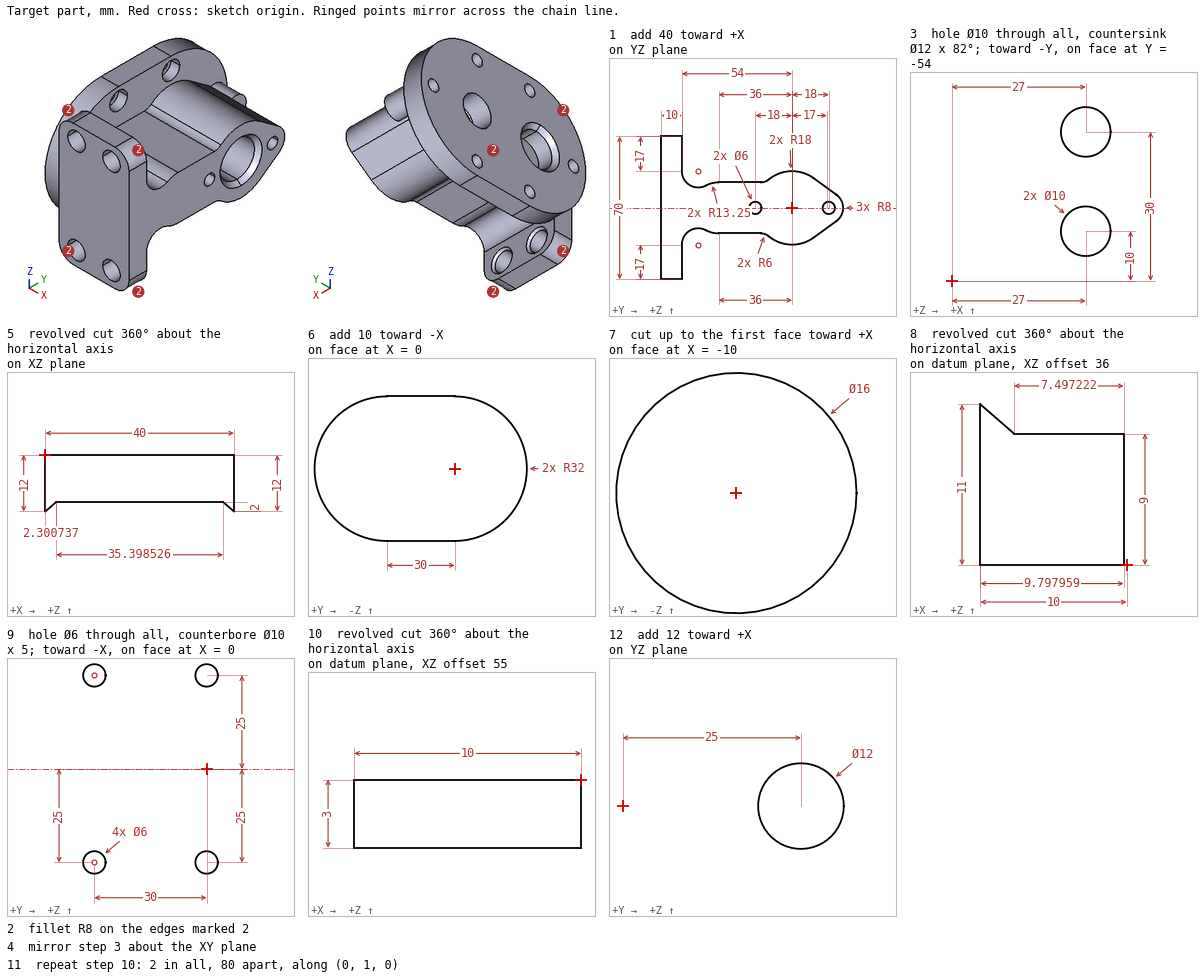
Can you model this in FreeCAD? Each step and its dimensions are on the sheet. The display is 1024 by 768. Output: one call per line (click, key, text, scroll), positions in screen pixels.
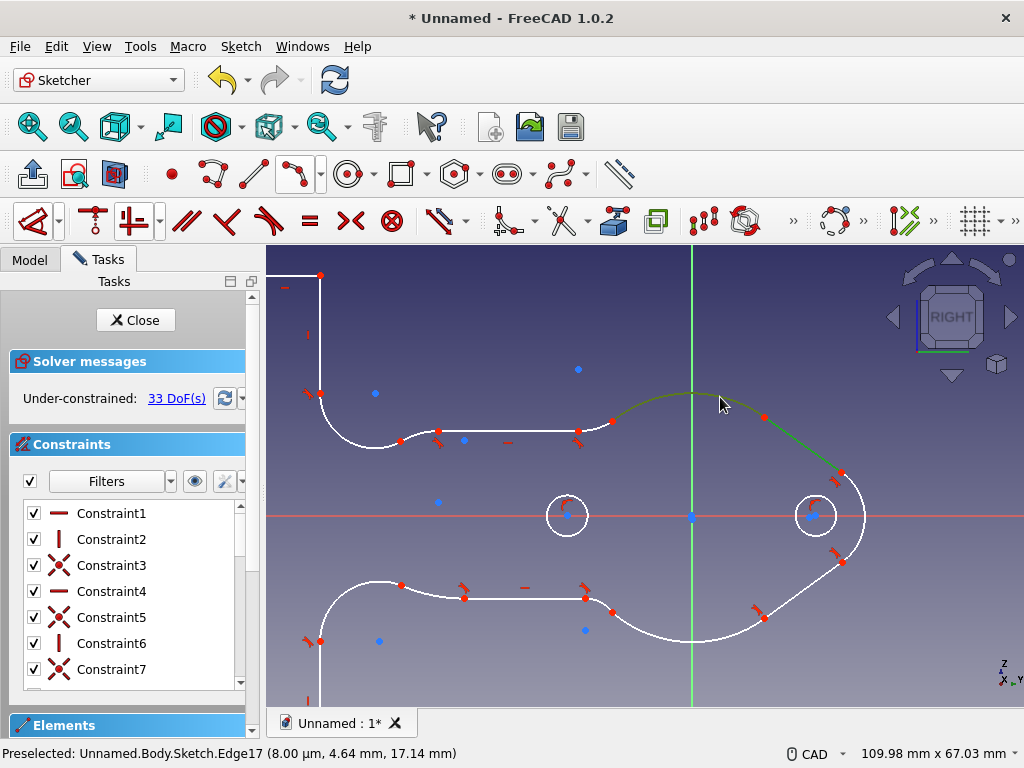
click(269, 222)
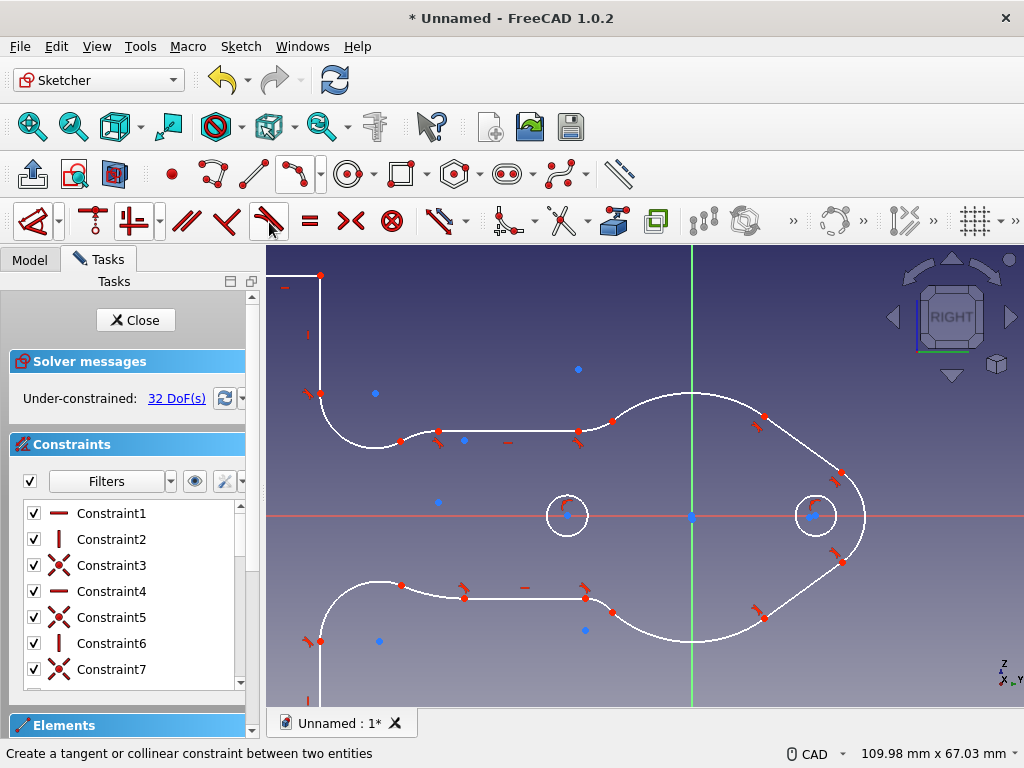
click(427, 432)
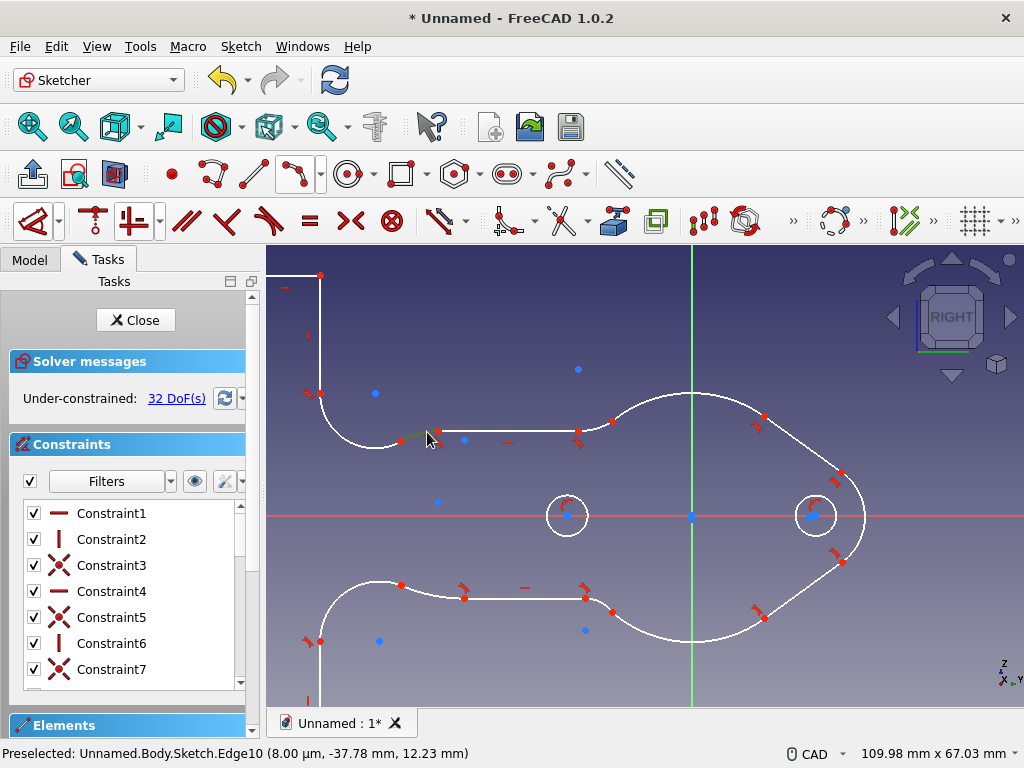
click(330, 425)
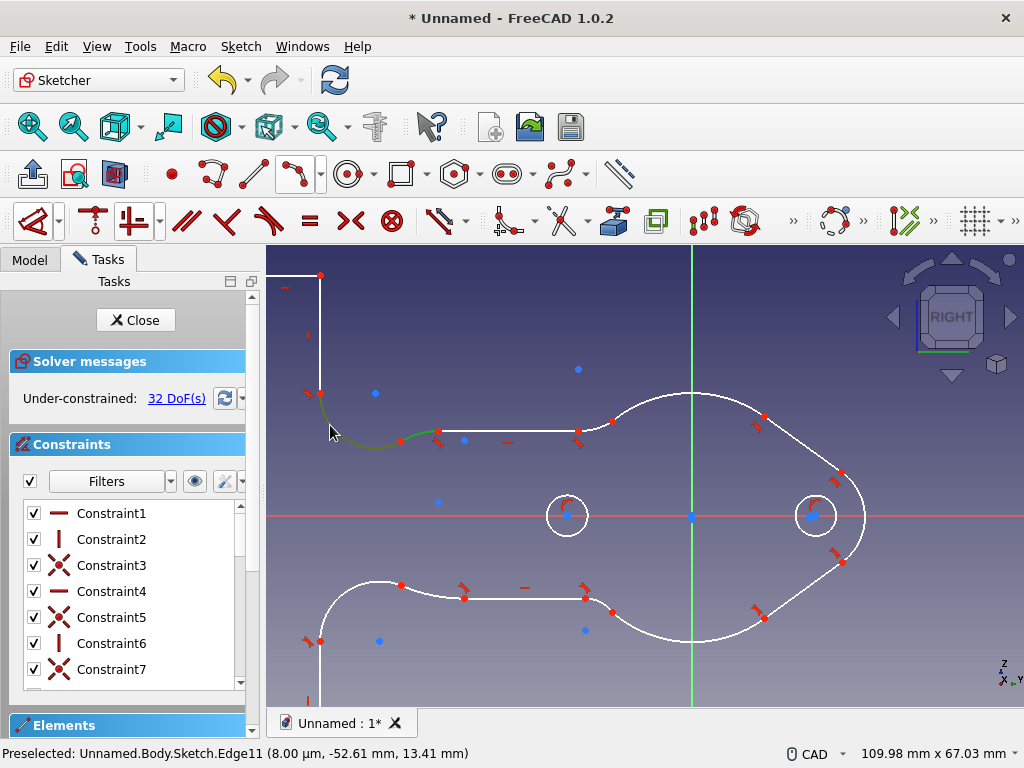
click(269, 222)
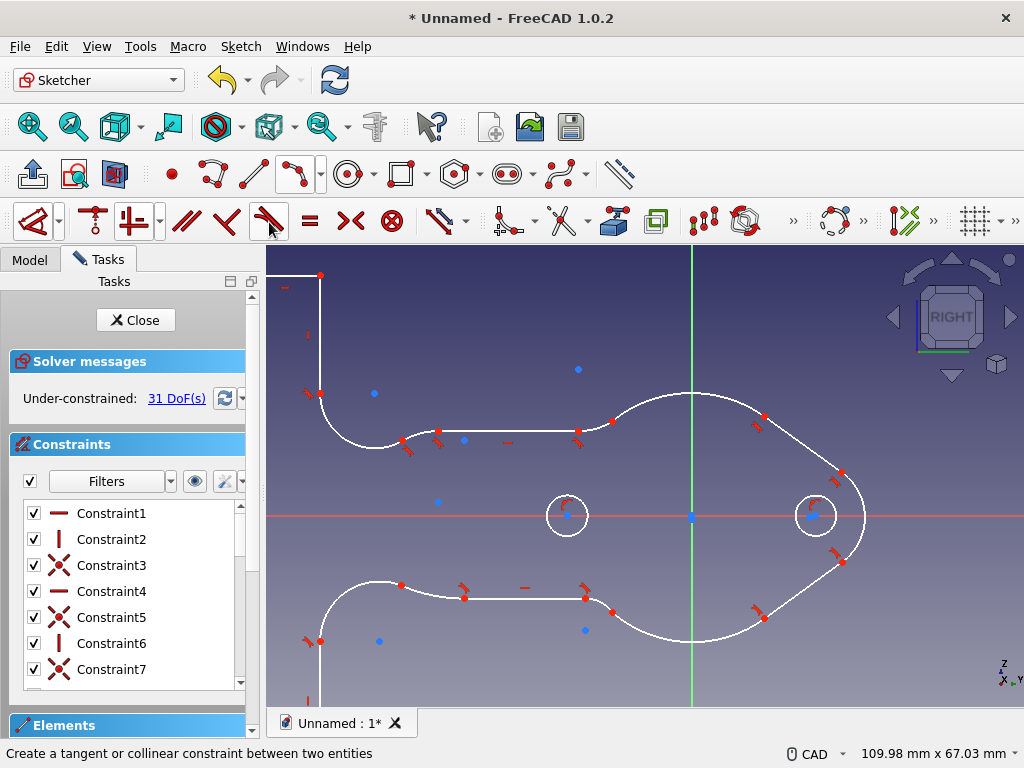
click(367, 583)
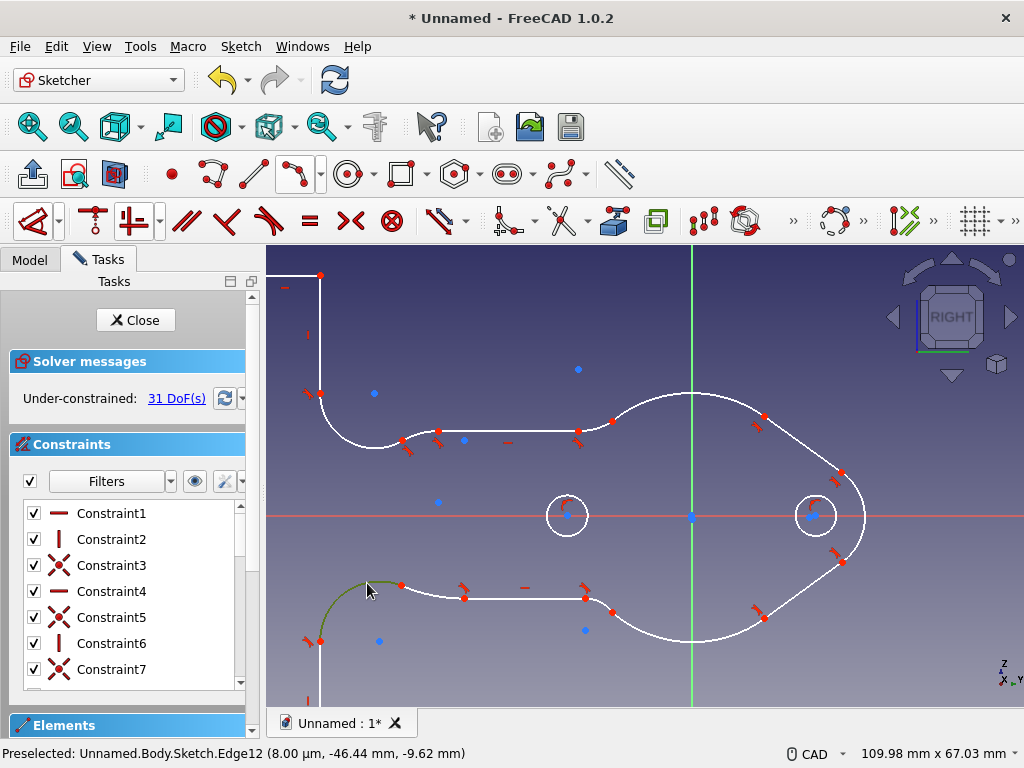
click(419, 592)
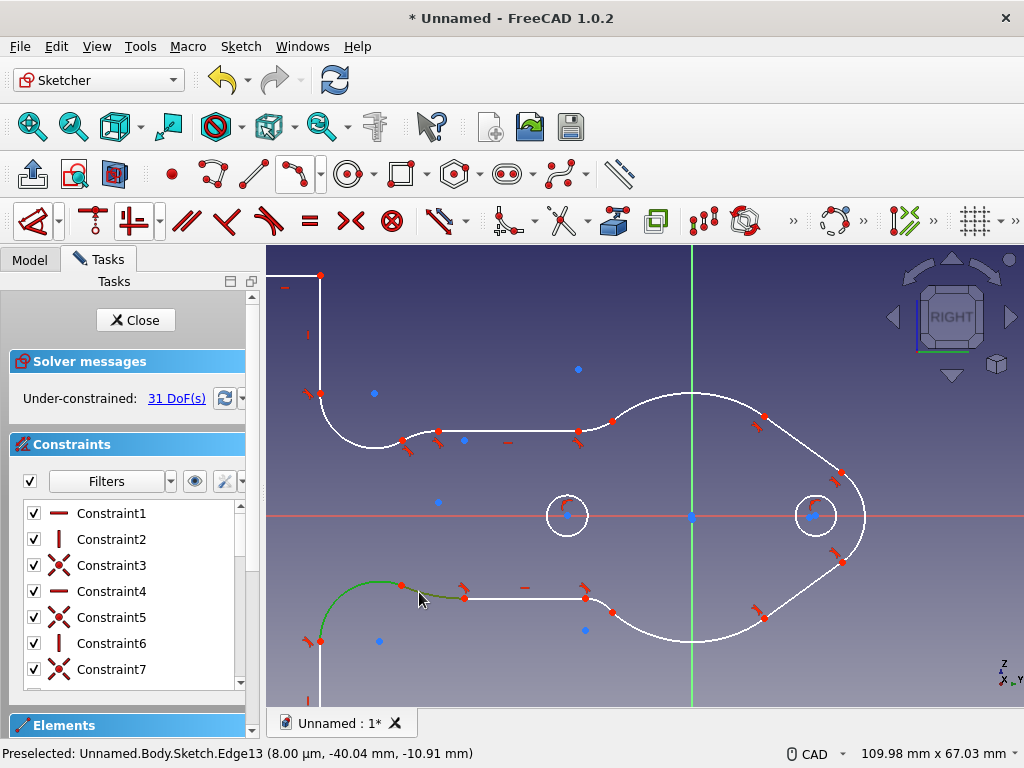
click(269, 222)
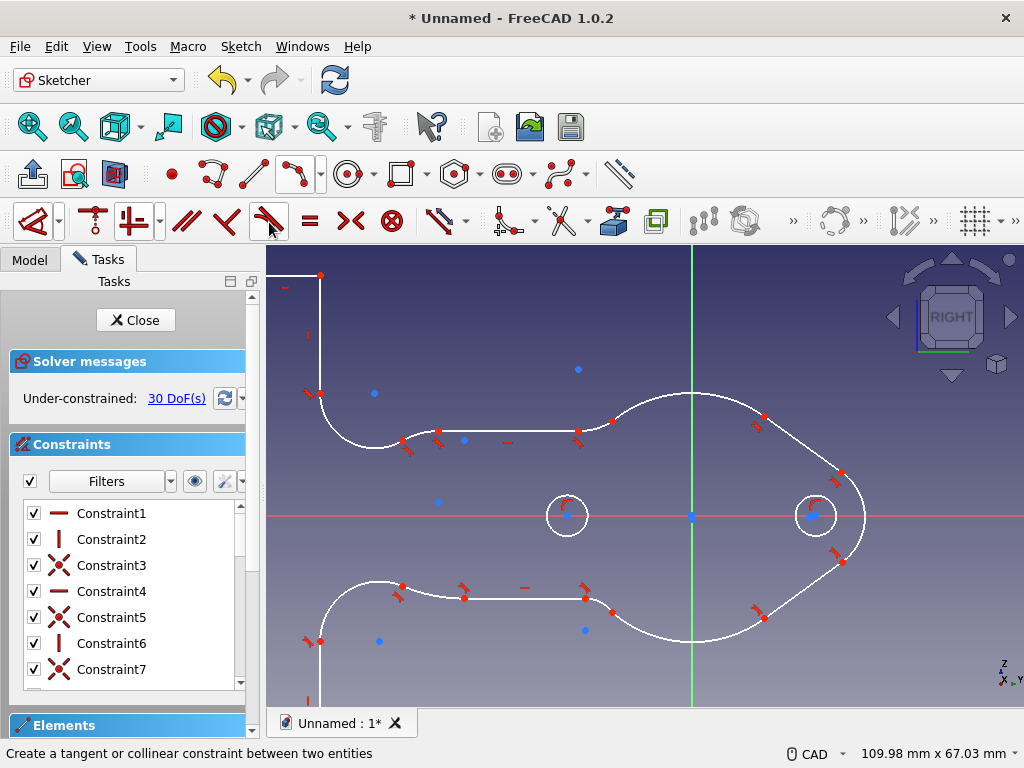
scroll(606, 606, up, 2)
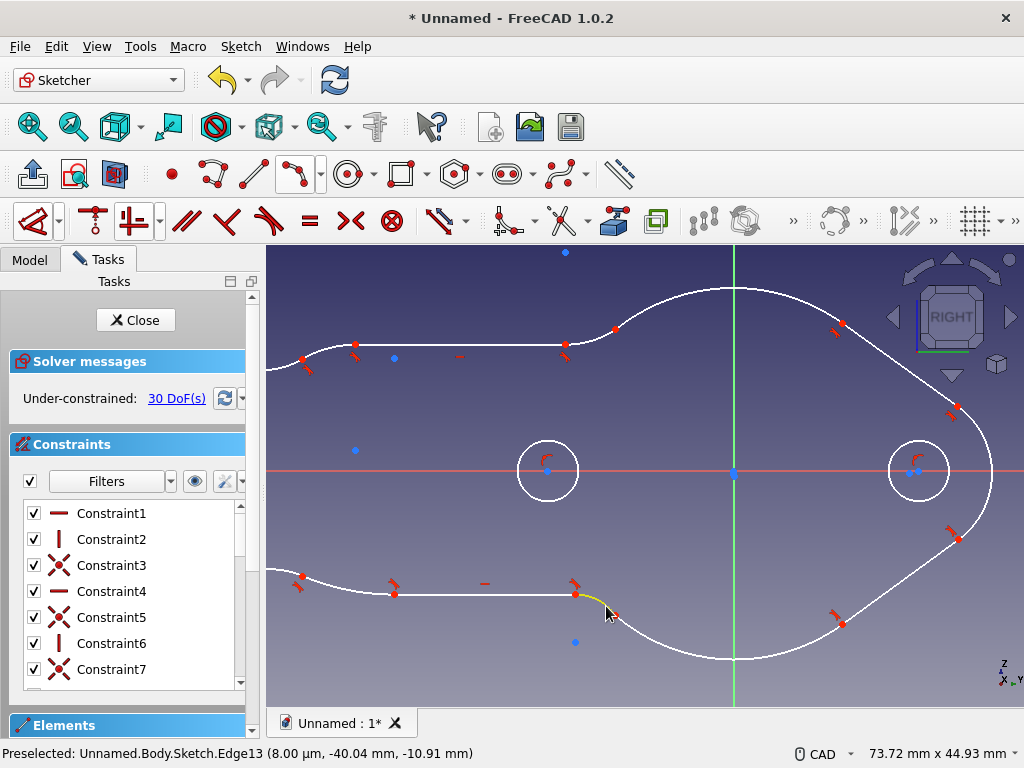
click(606, 605)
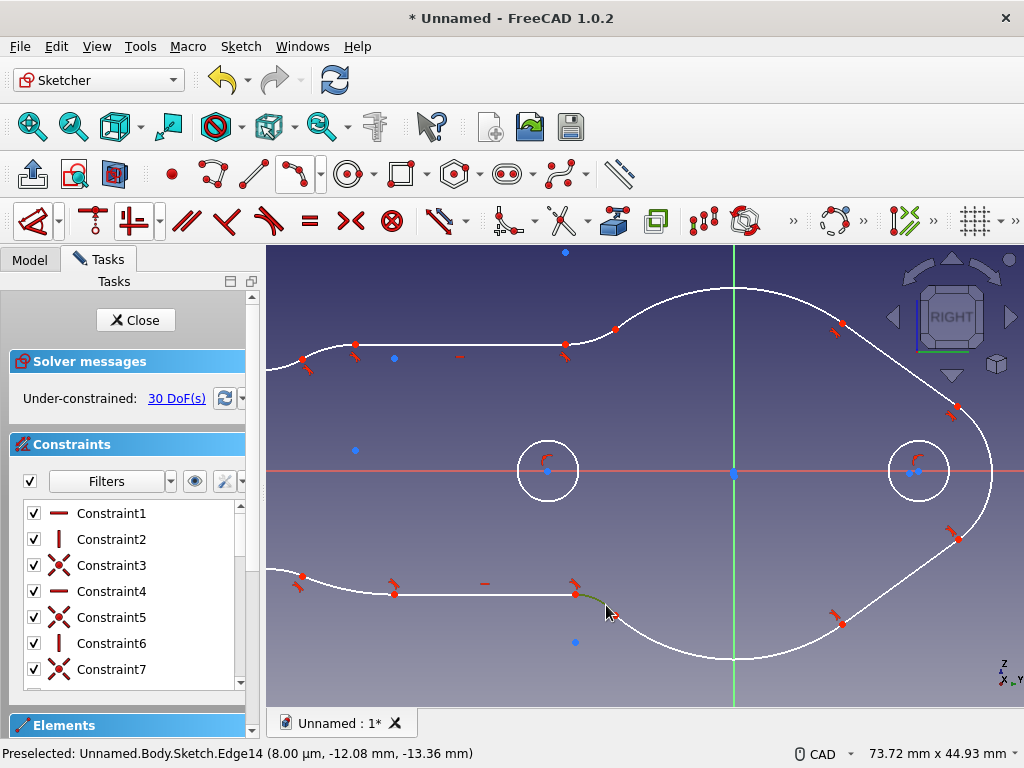
click(679, 651)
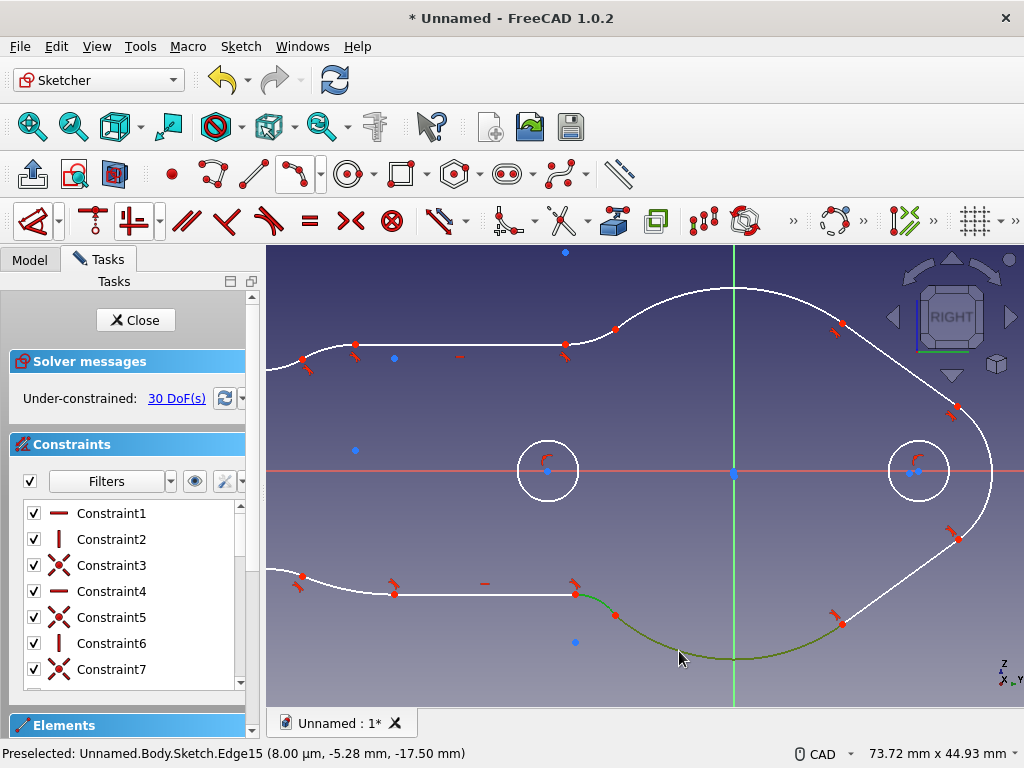
click(269, 222)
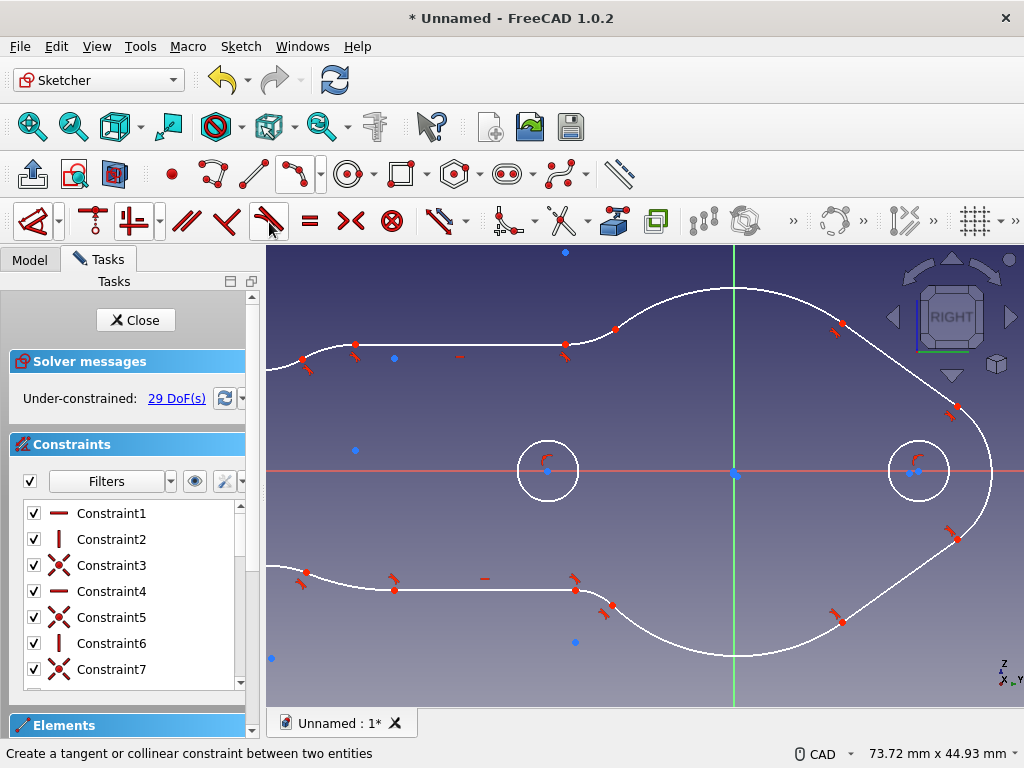
click(776, 293)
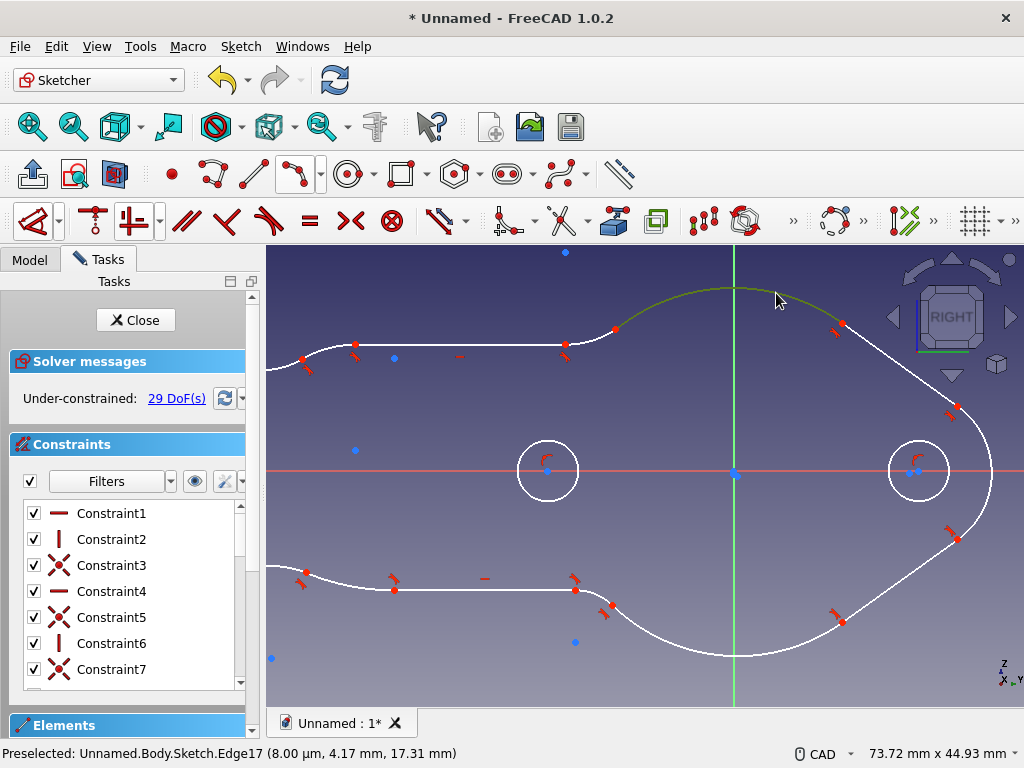
click(581, 343)